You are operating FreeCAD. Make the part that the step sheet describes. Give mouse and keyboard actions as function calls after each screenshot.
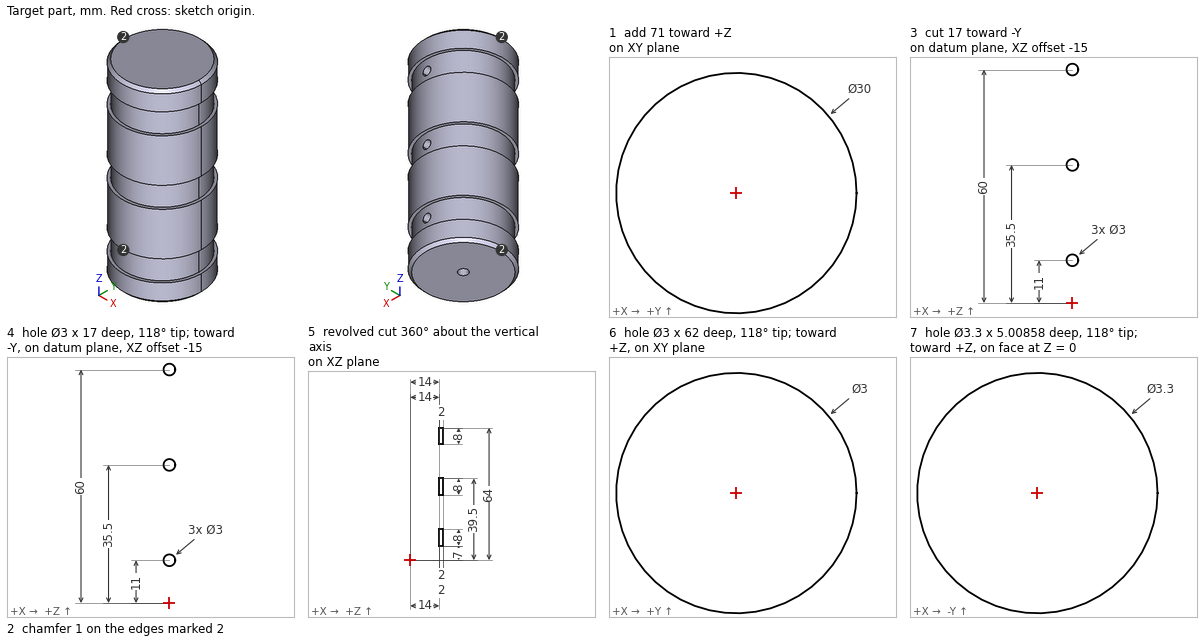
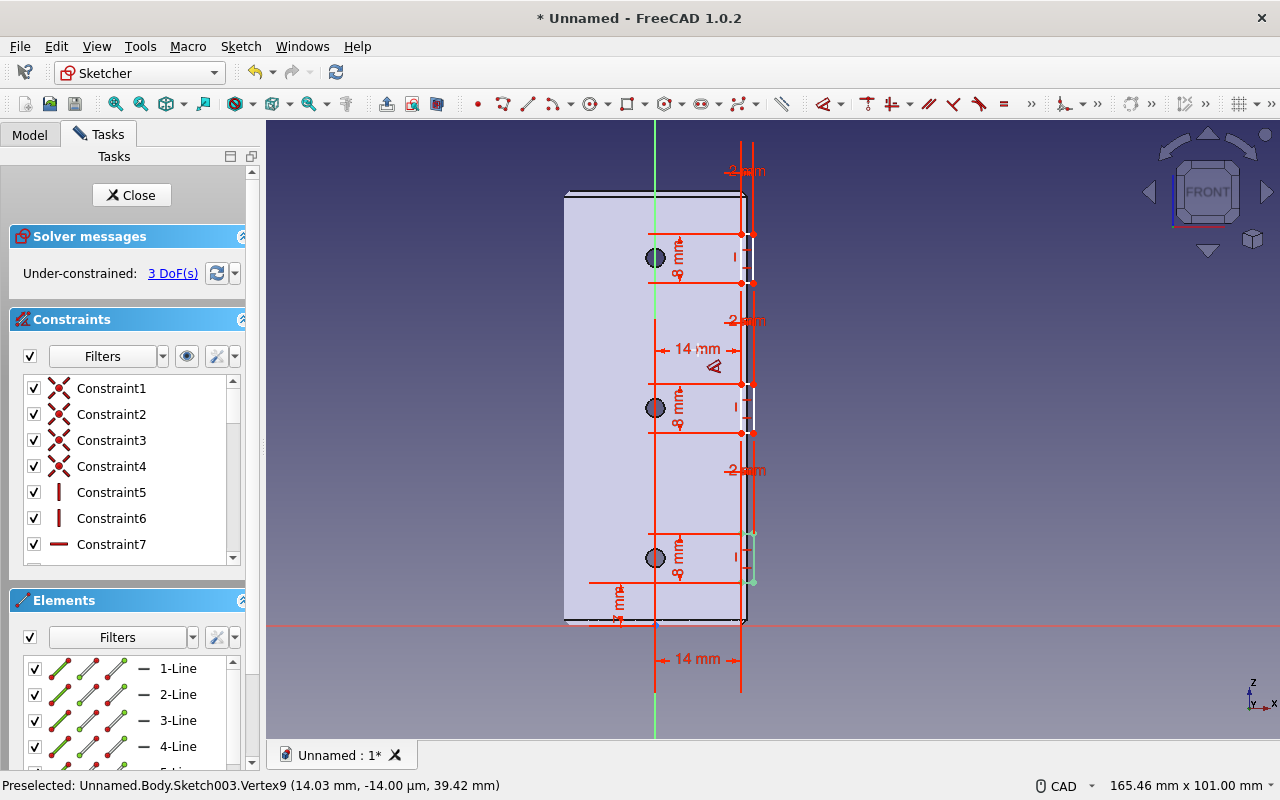
click(741, 234)
click(698, 200)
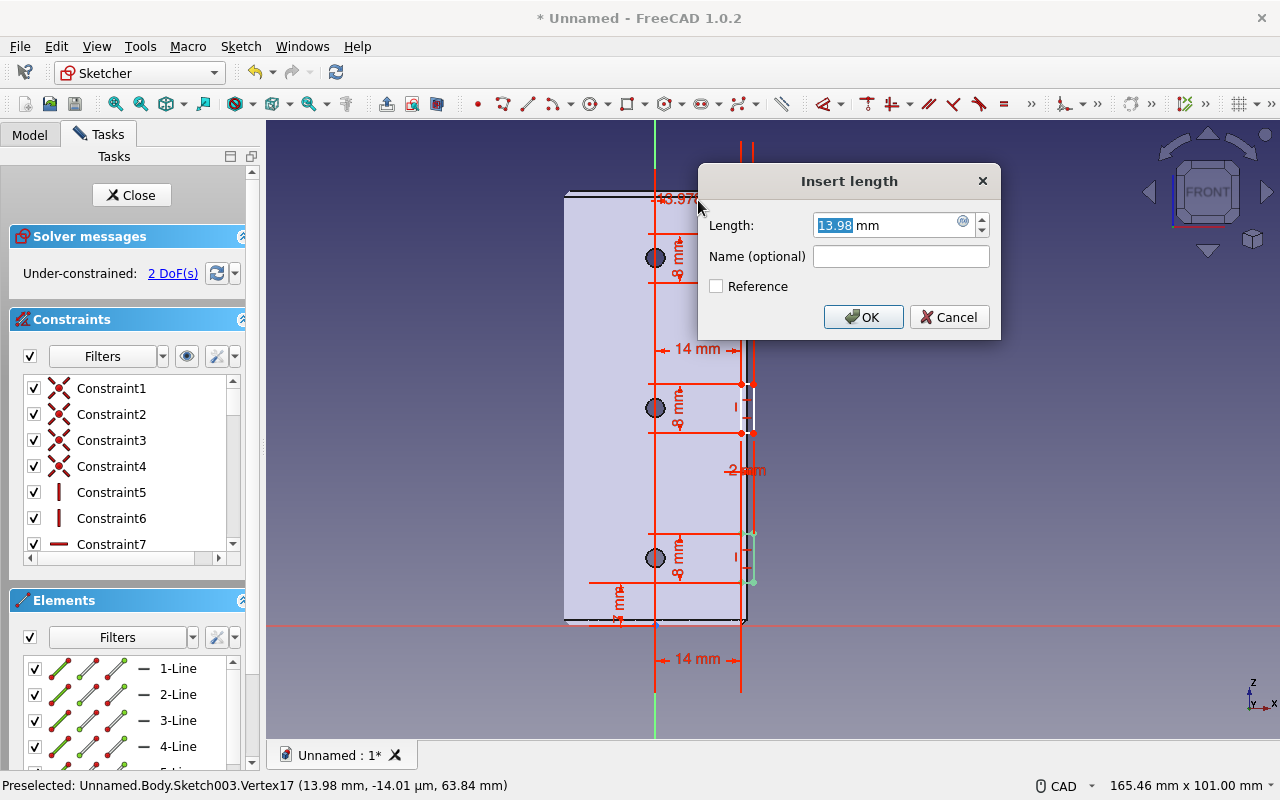
text(14)
key(Return)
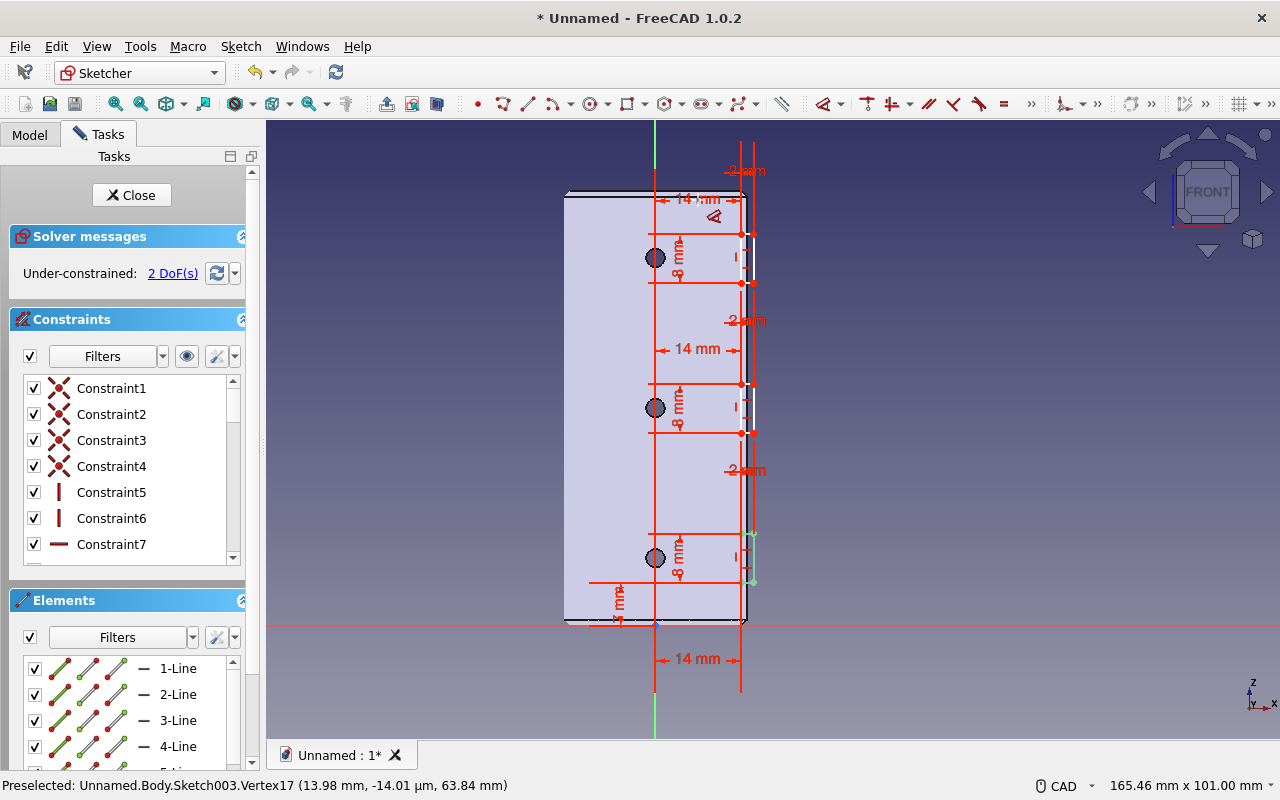
click(741, 234)
click(621, 430)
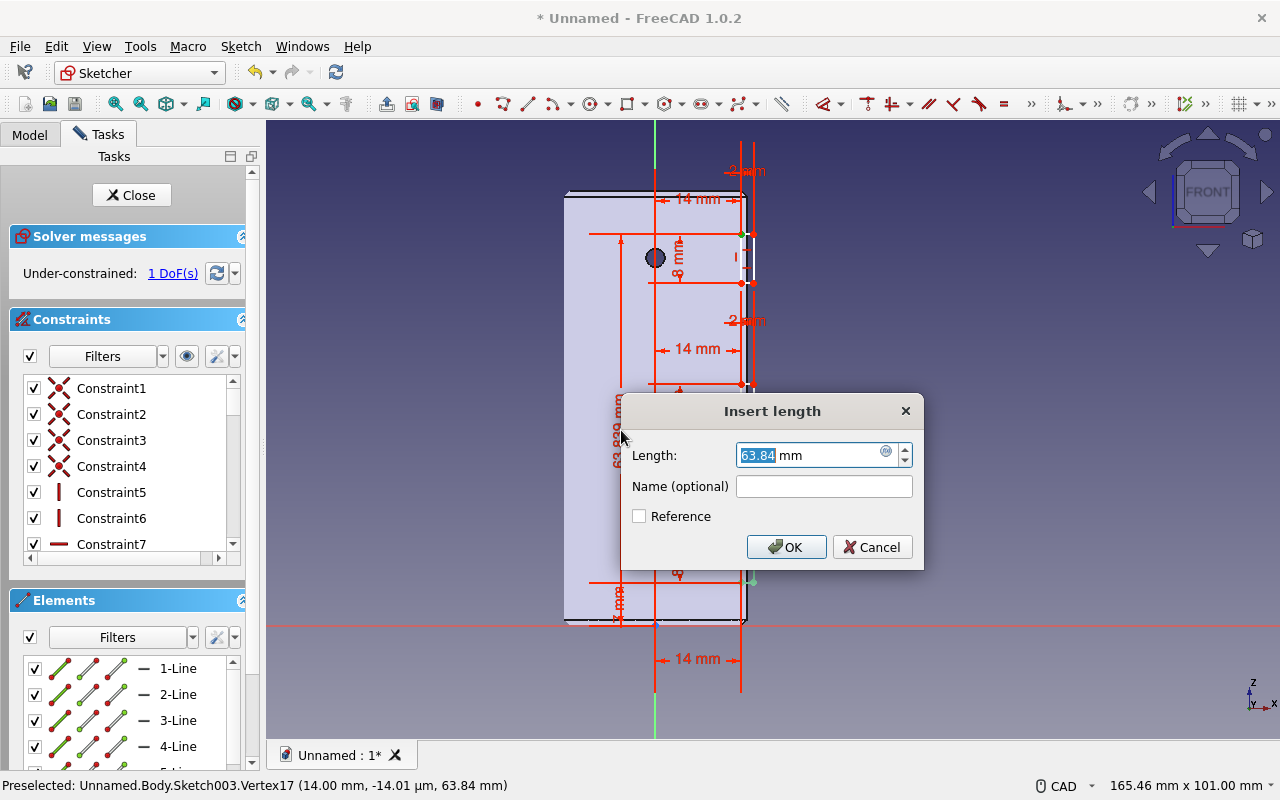
text(64)
key(Return)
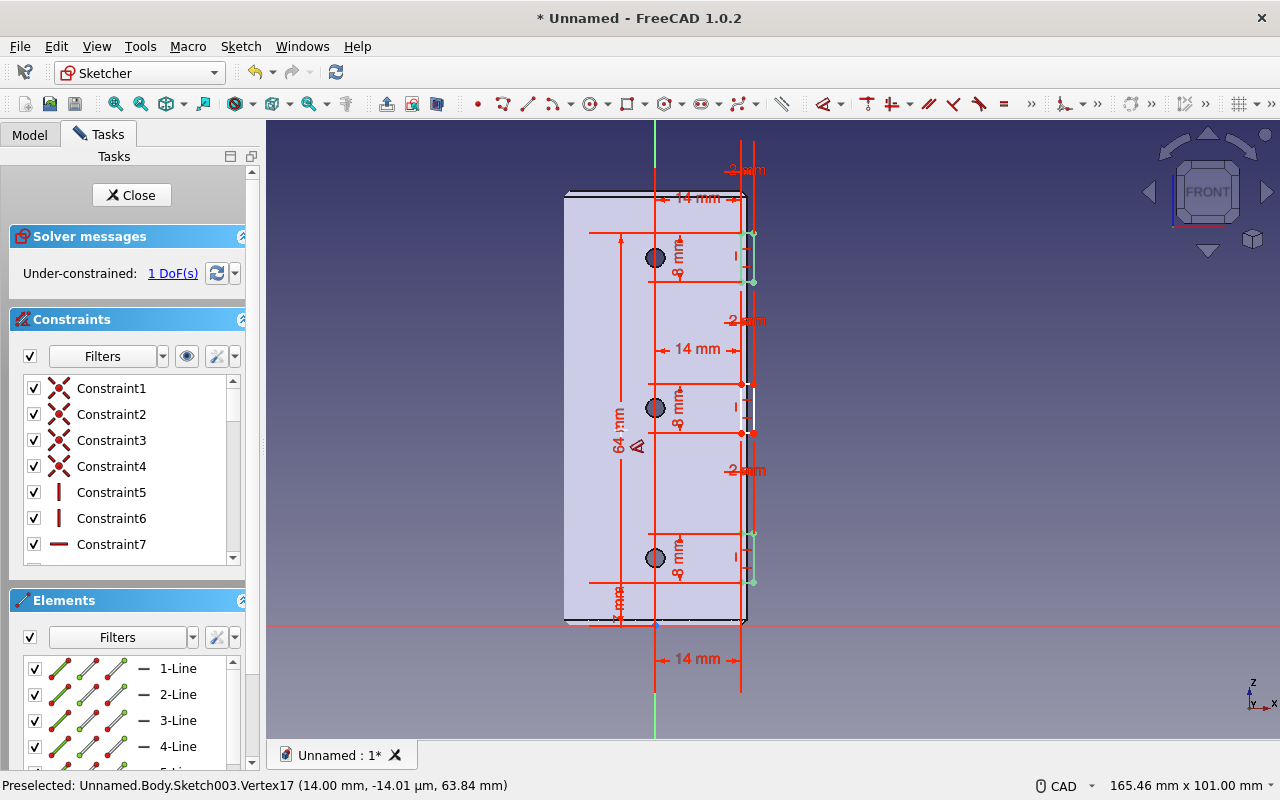
click(741, 384)
click(621, 505)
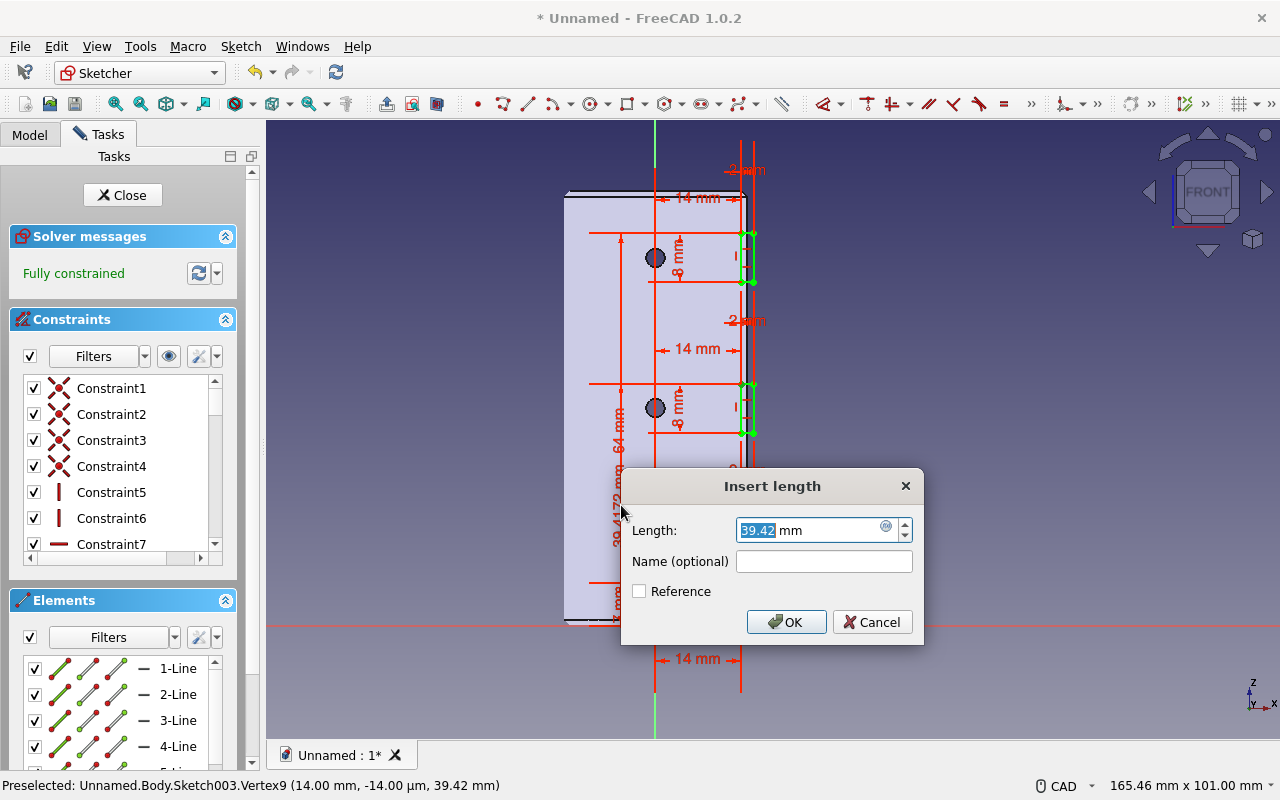
text(39.5)
key(Return)
key(Escape)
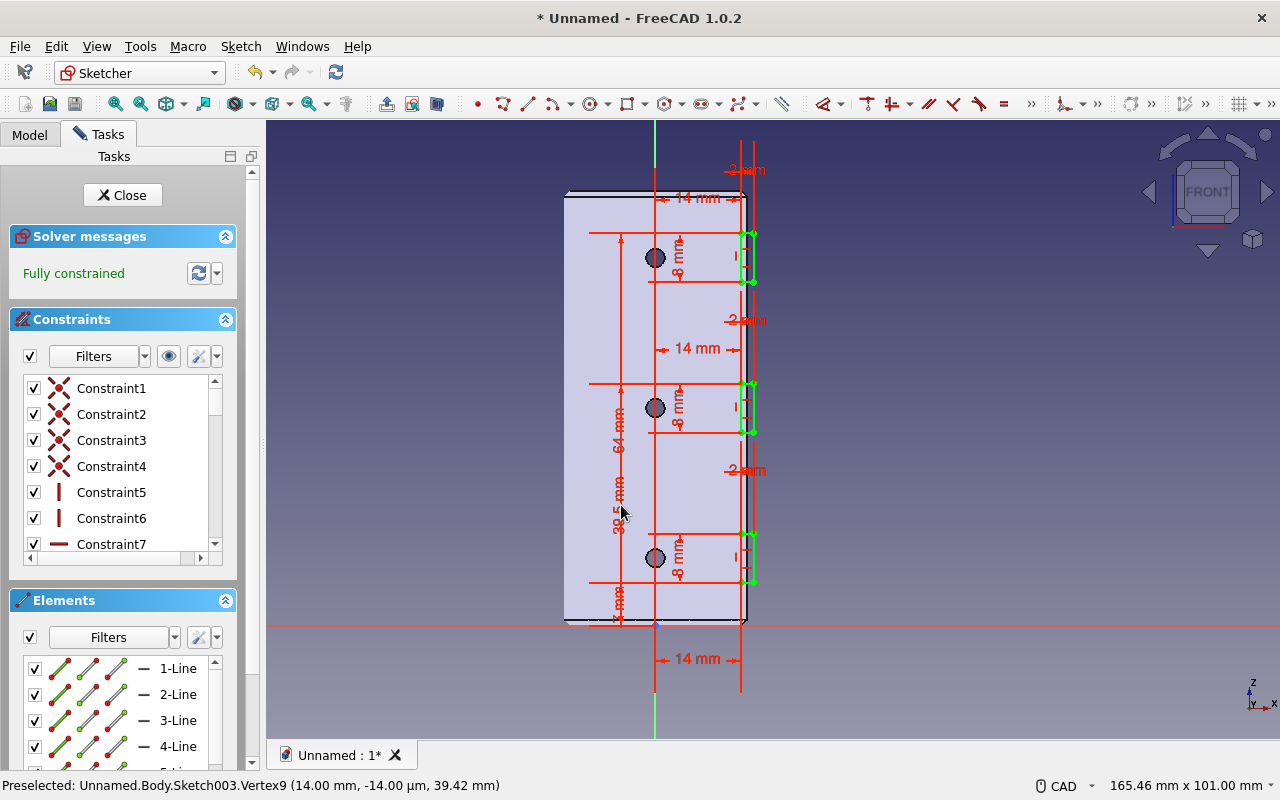
click(123, 195)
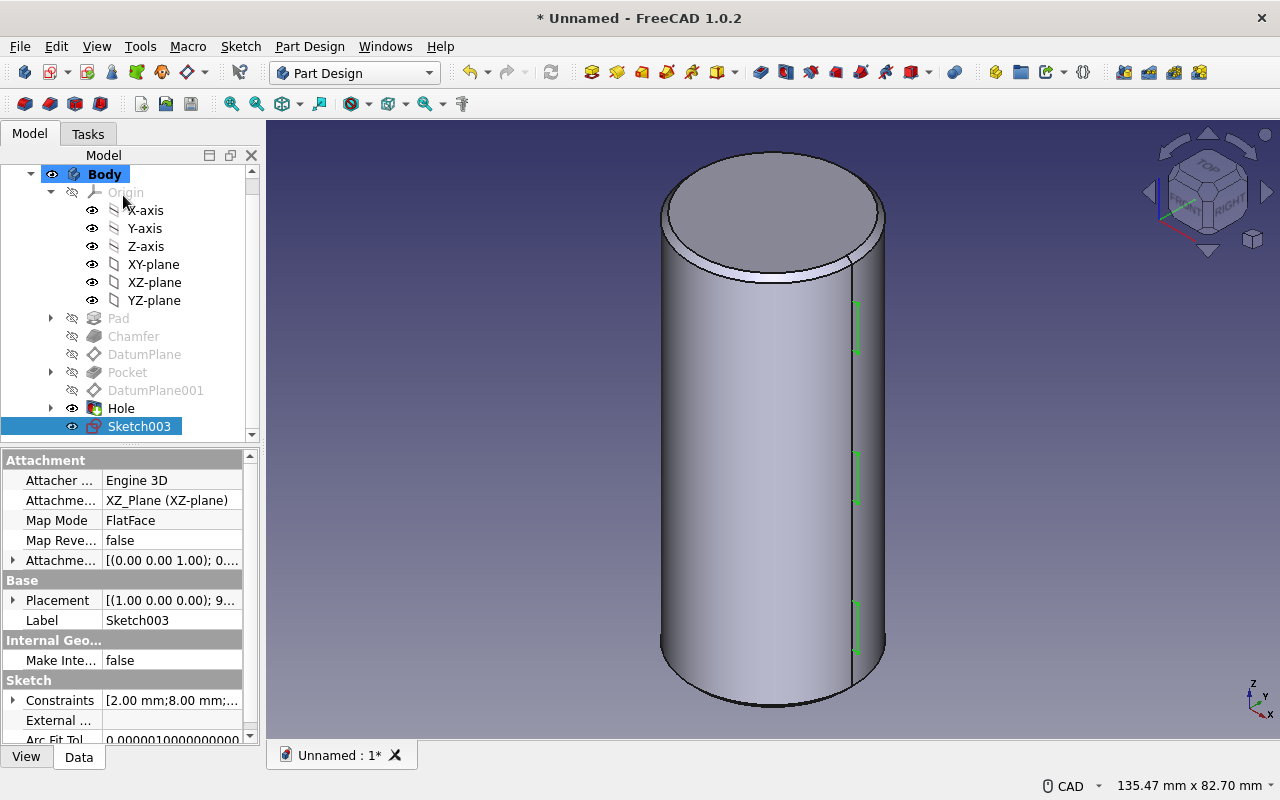
click(811, 72)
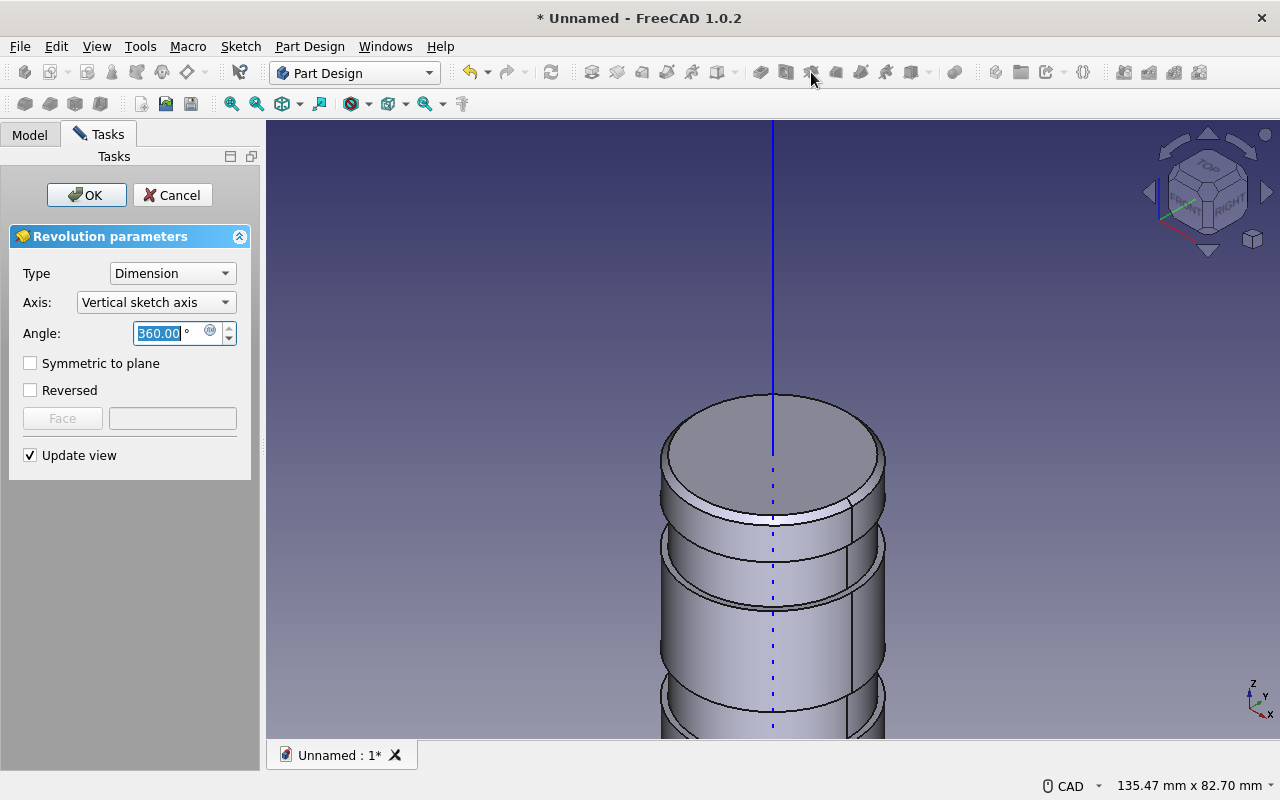
click(87, 195)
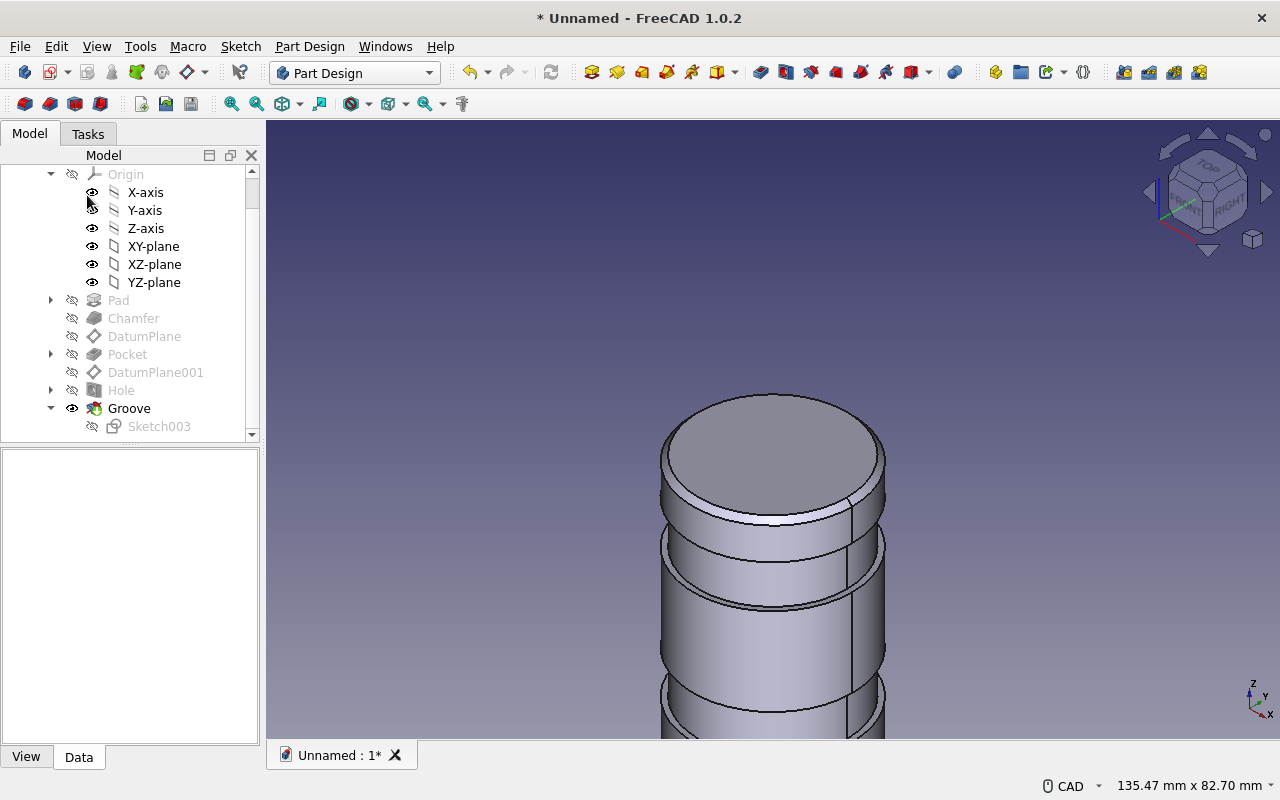
click(232, 104)